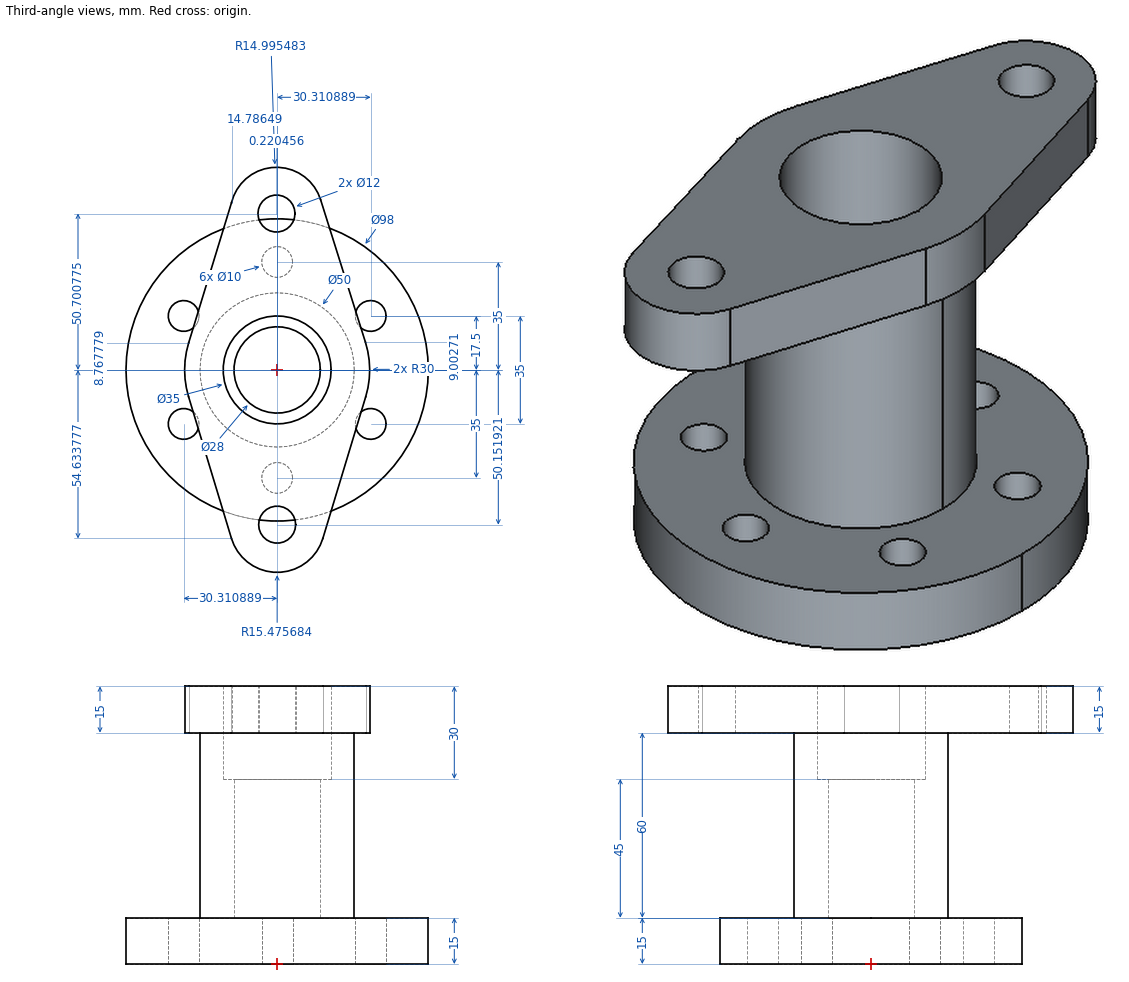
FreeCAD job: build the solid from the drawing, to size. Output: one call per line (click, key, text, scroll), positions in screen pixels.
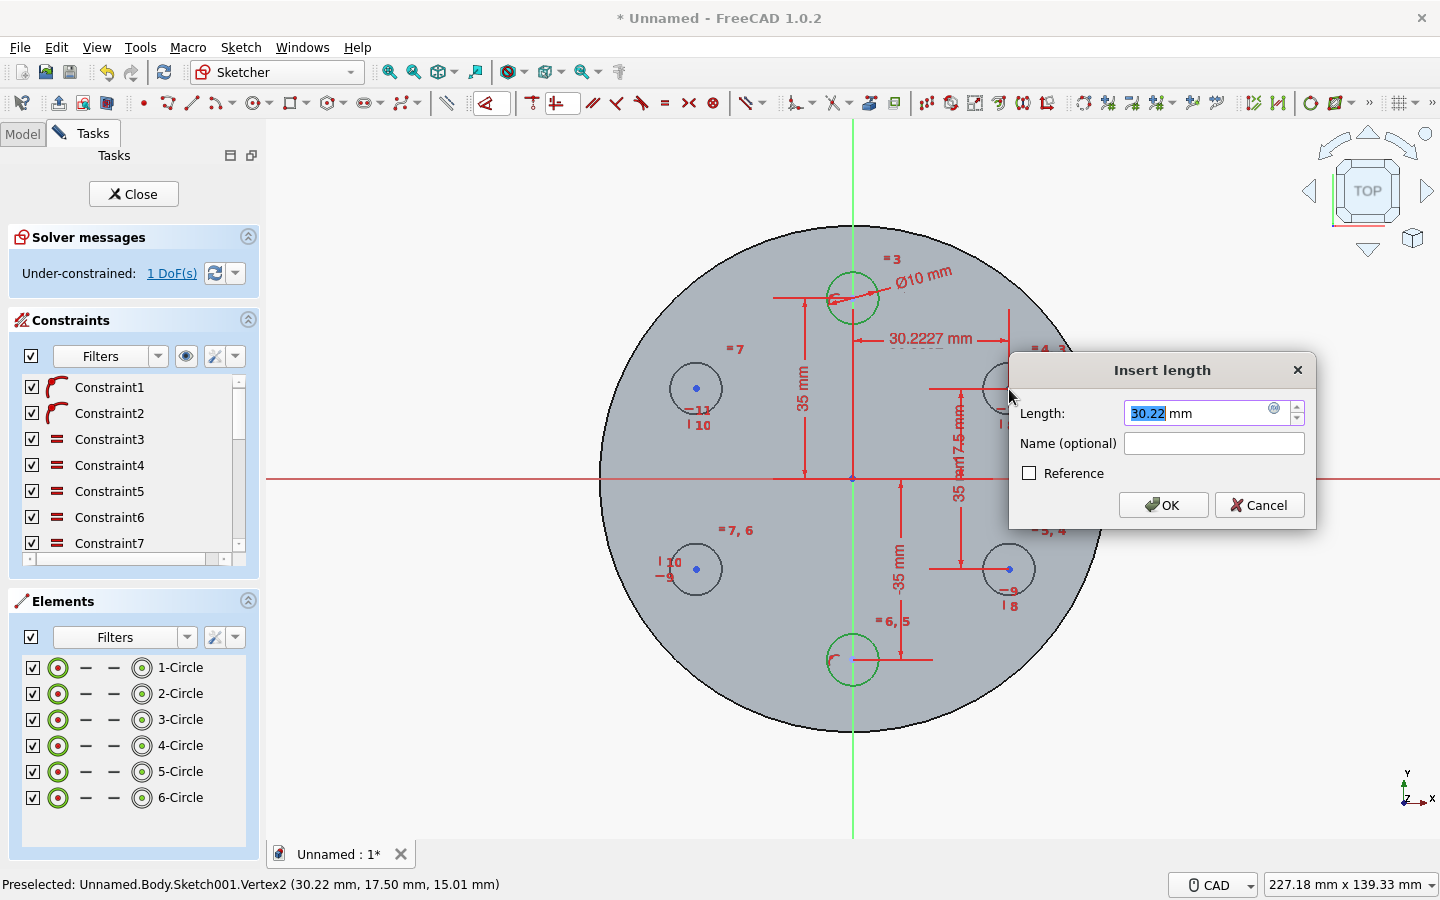
text(30.310889)
key(Return)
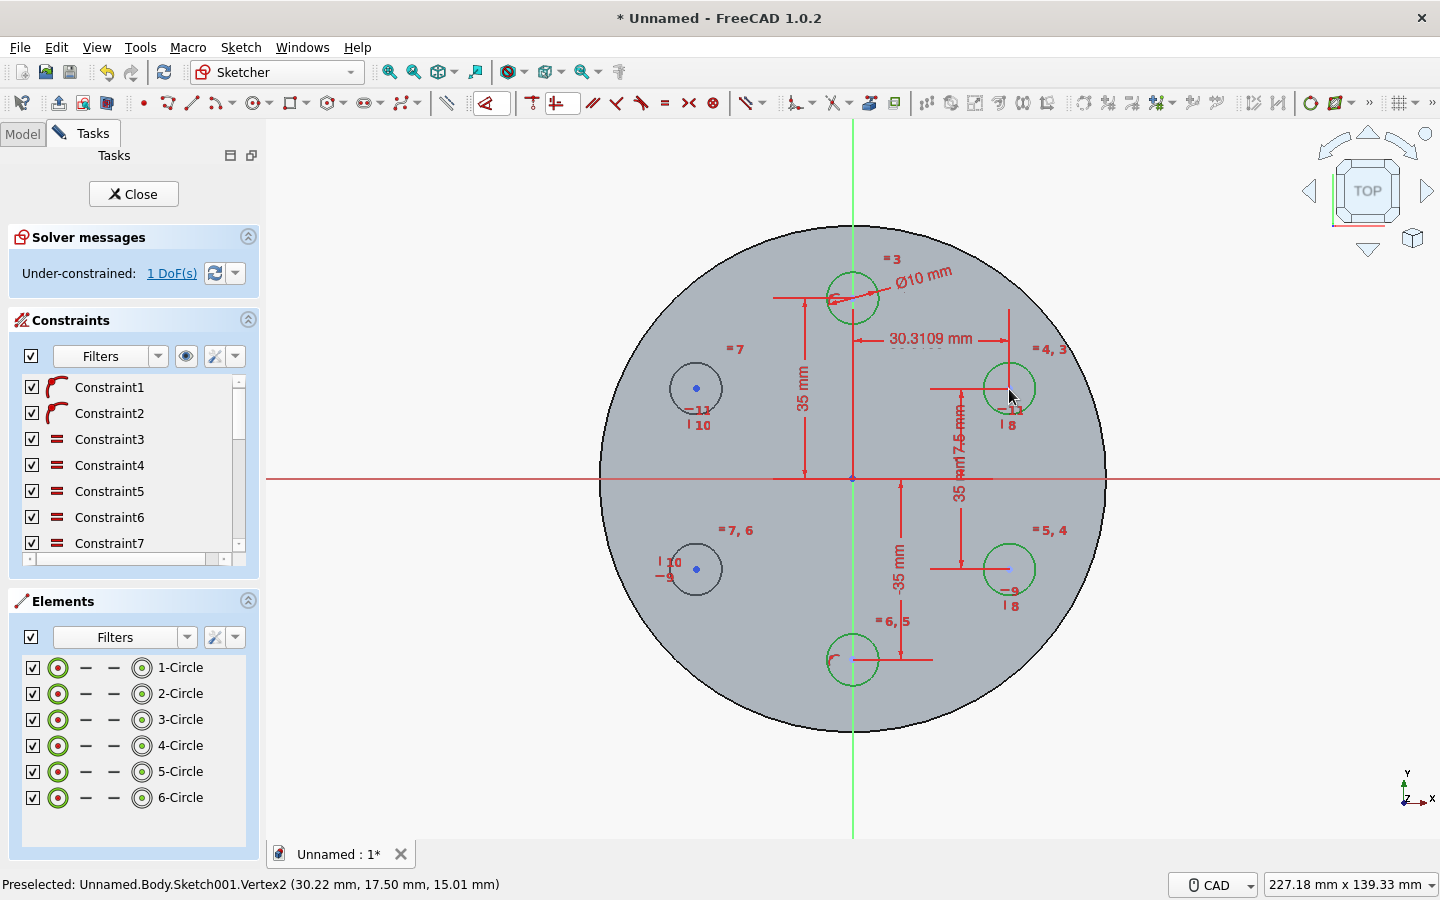
click(696, 569)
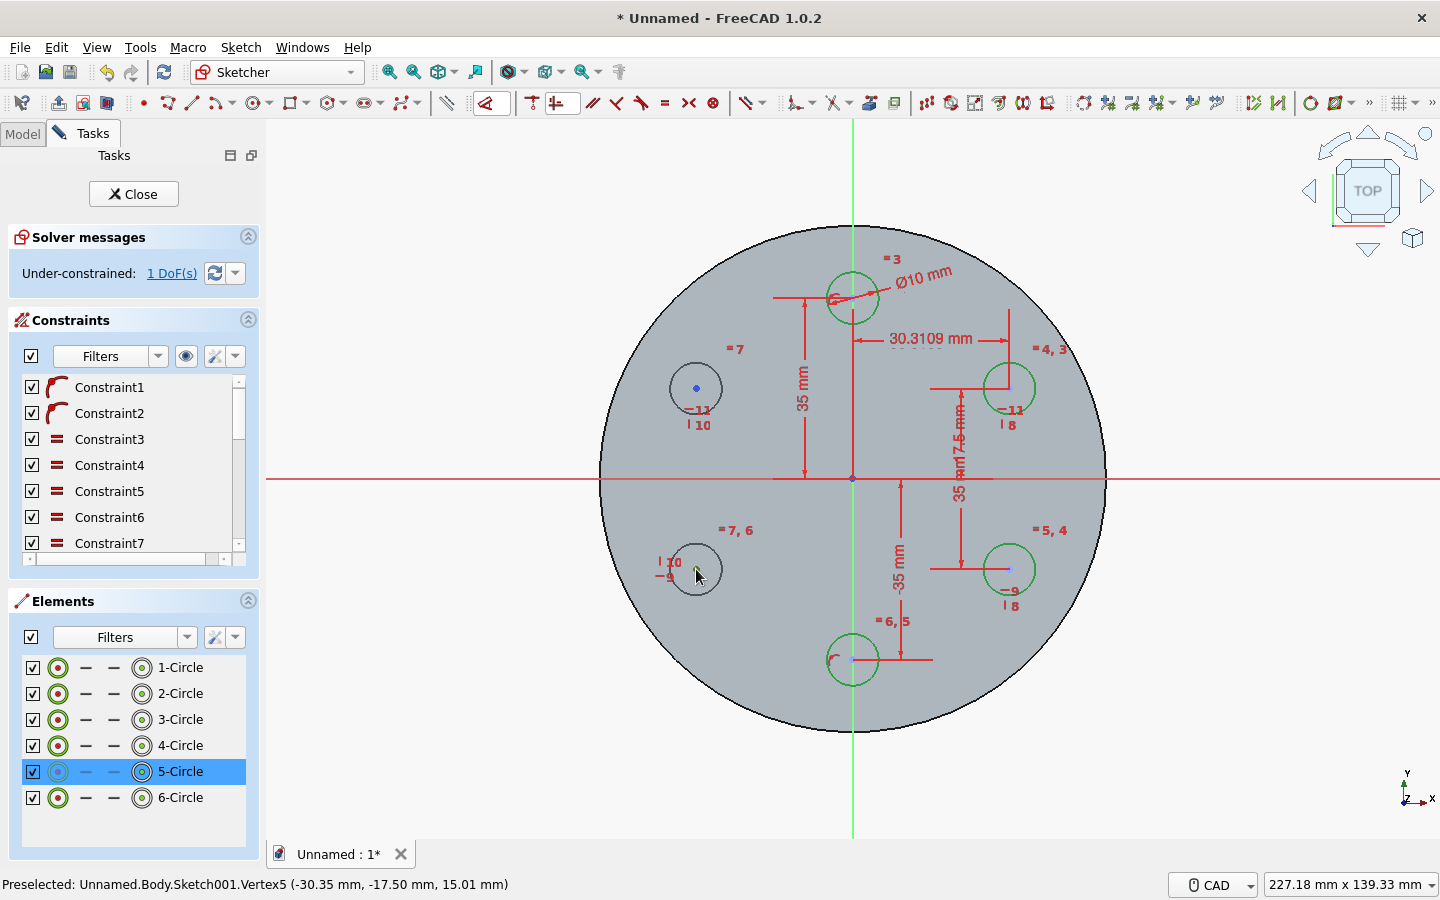
click(504, 104)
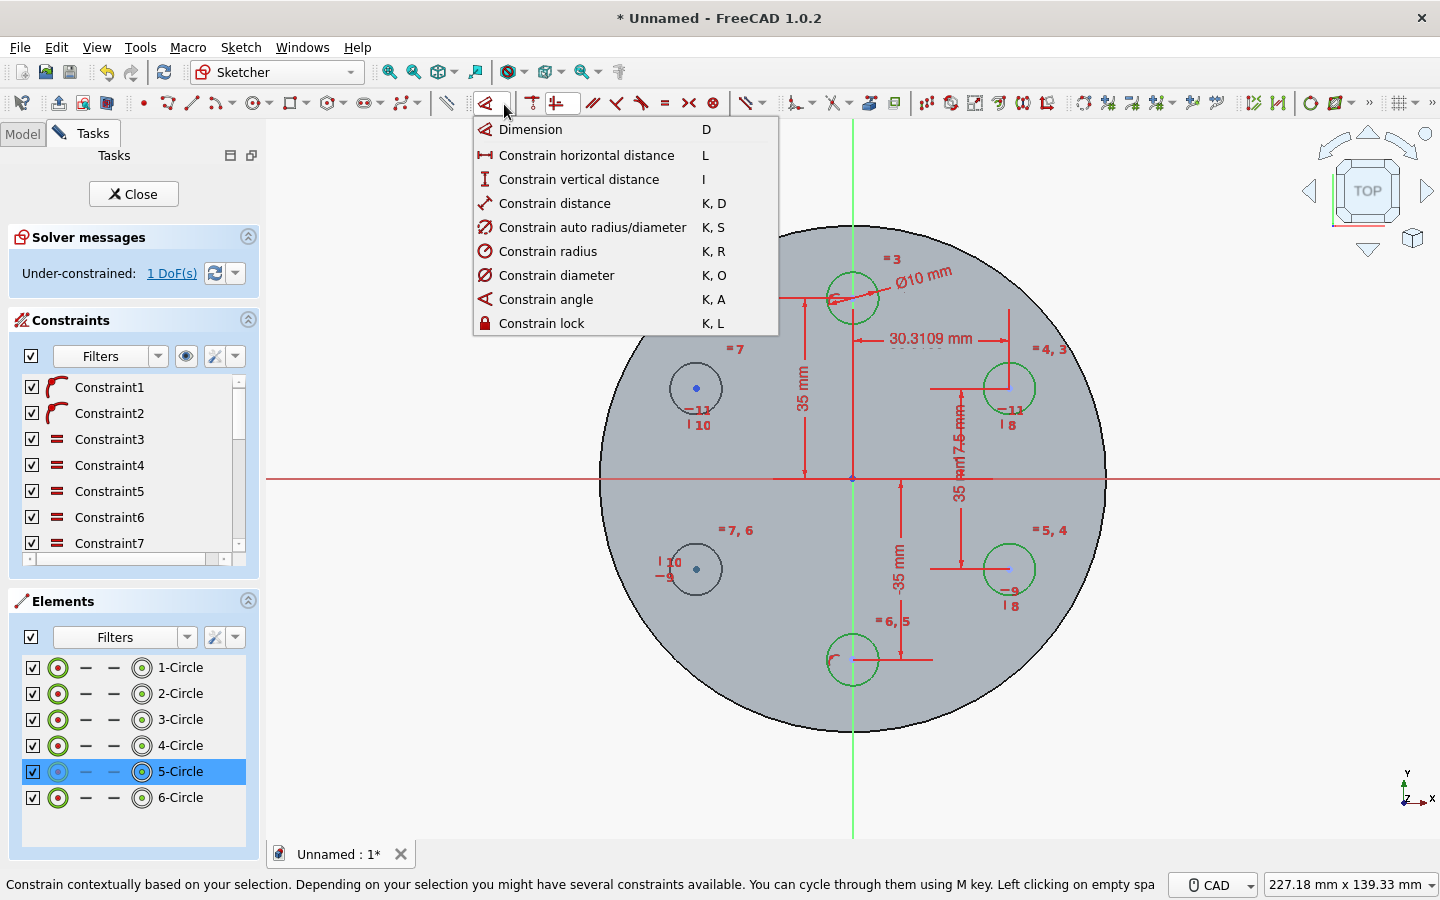
click(626, 155)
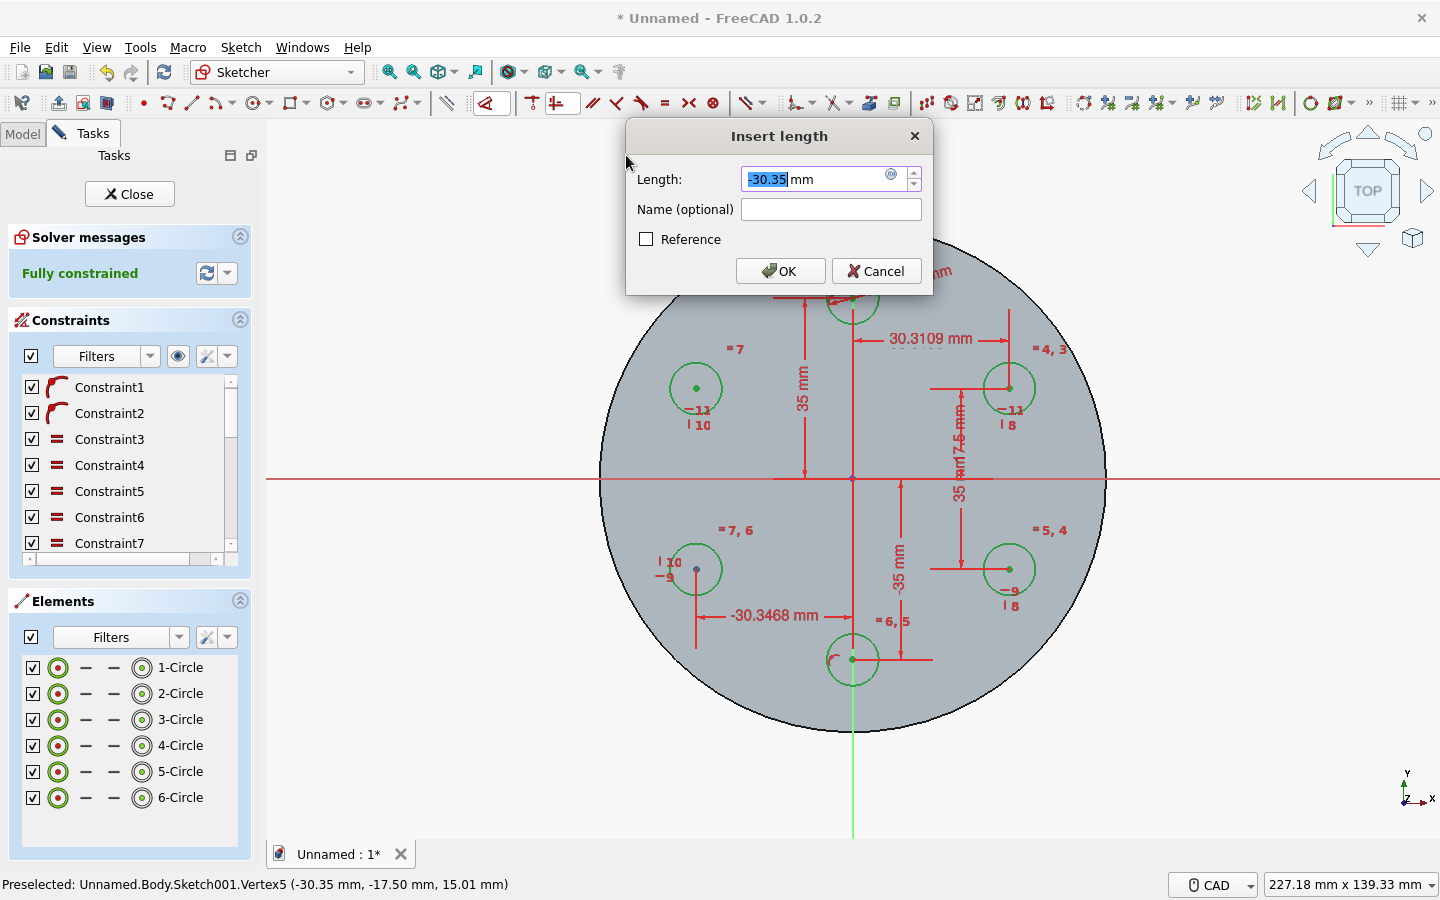
text(-30.310889)
key(Return)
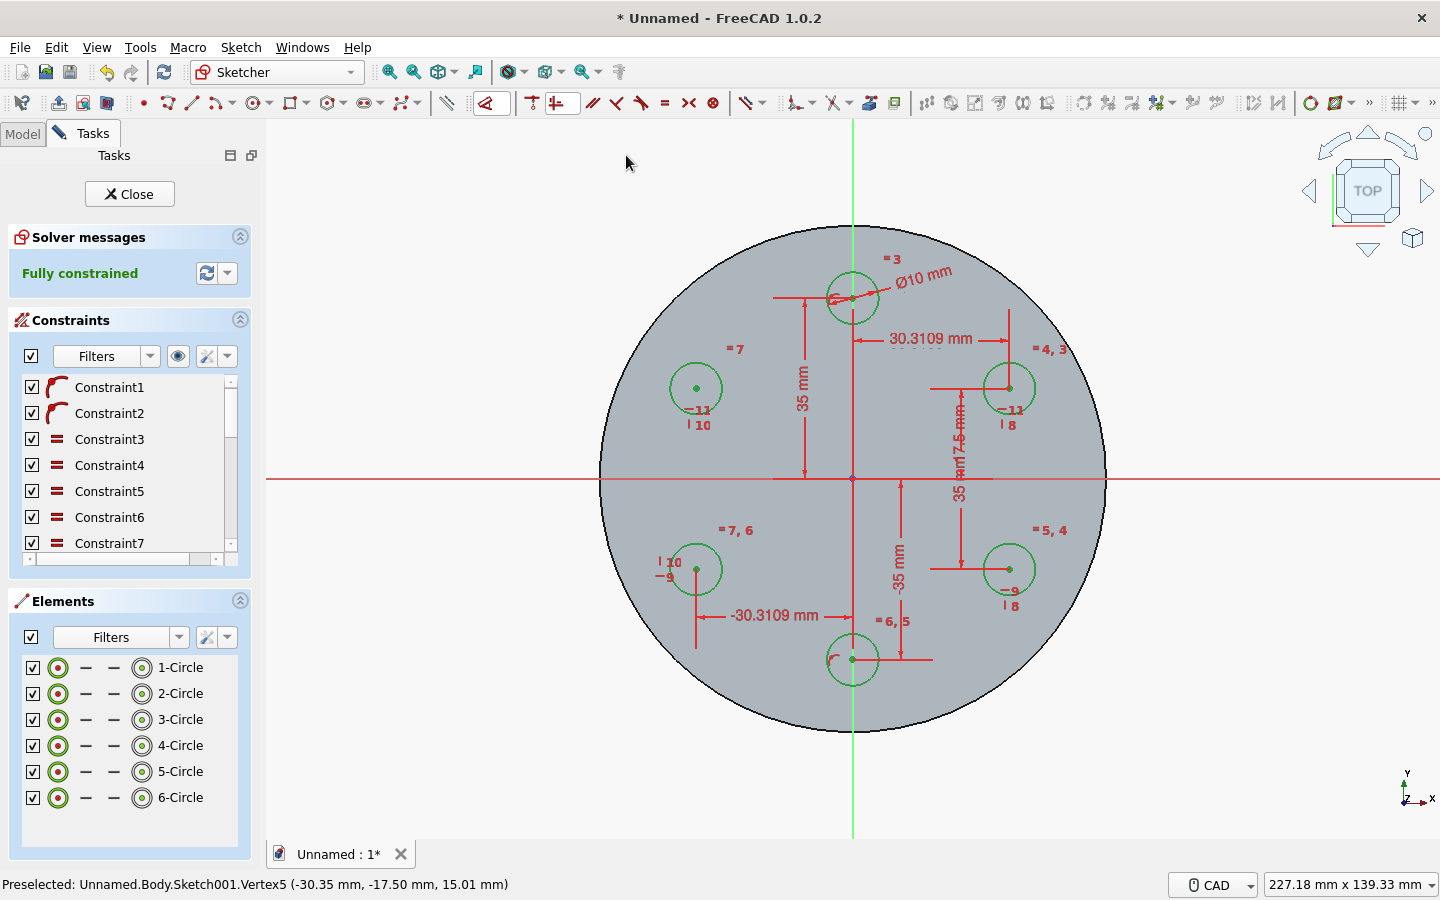
click(130, 194)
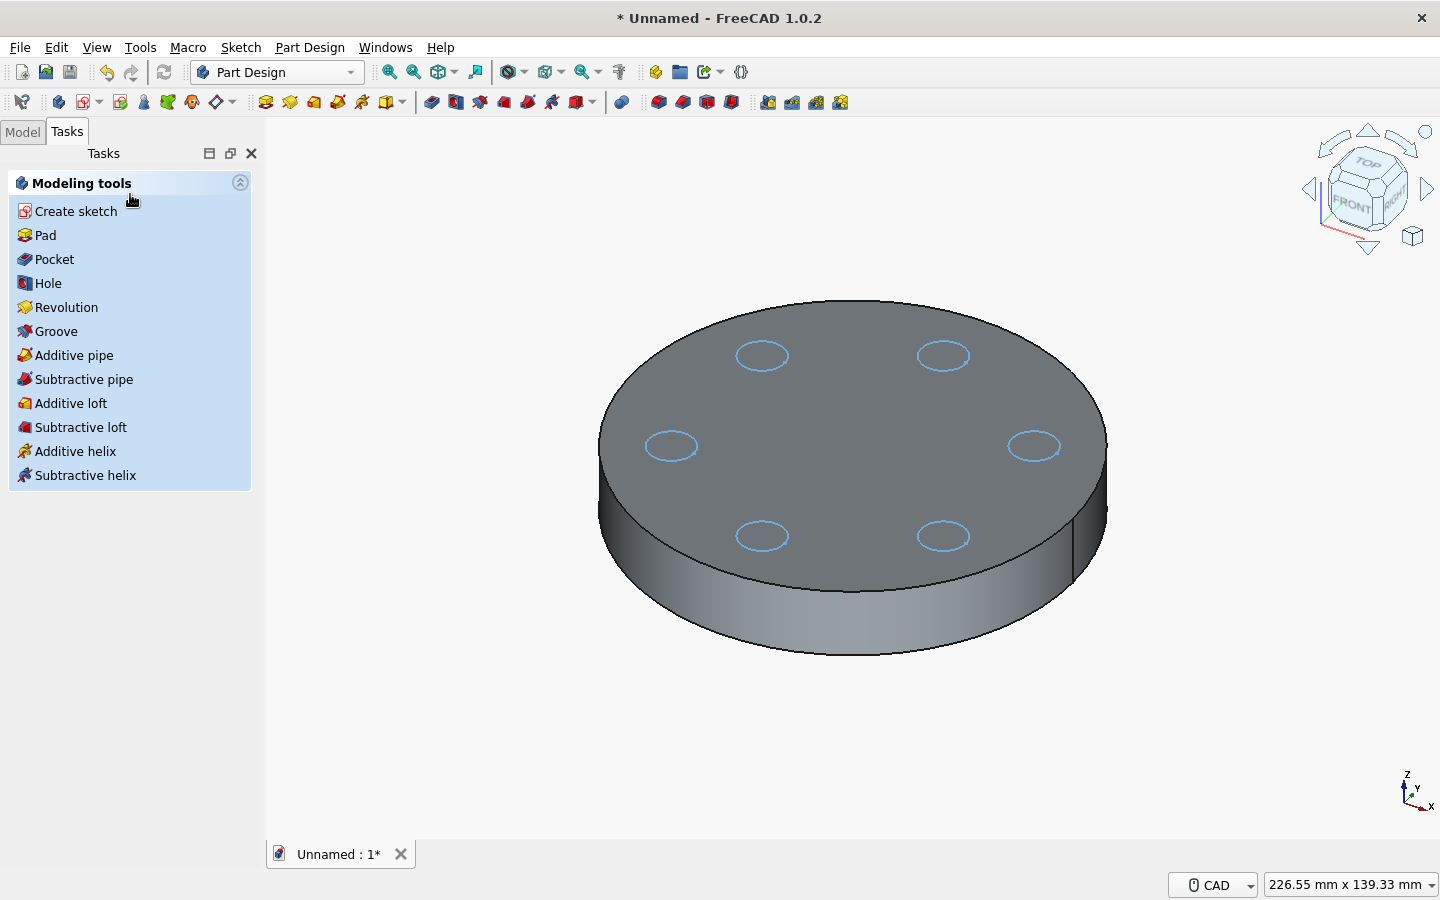
click(432, 102)